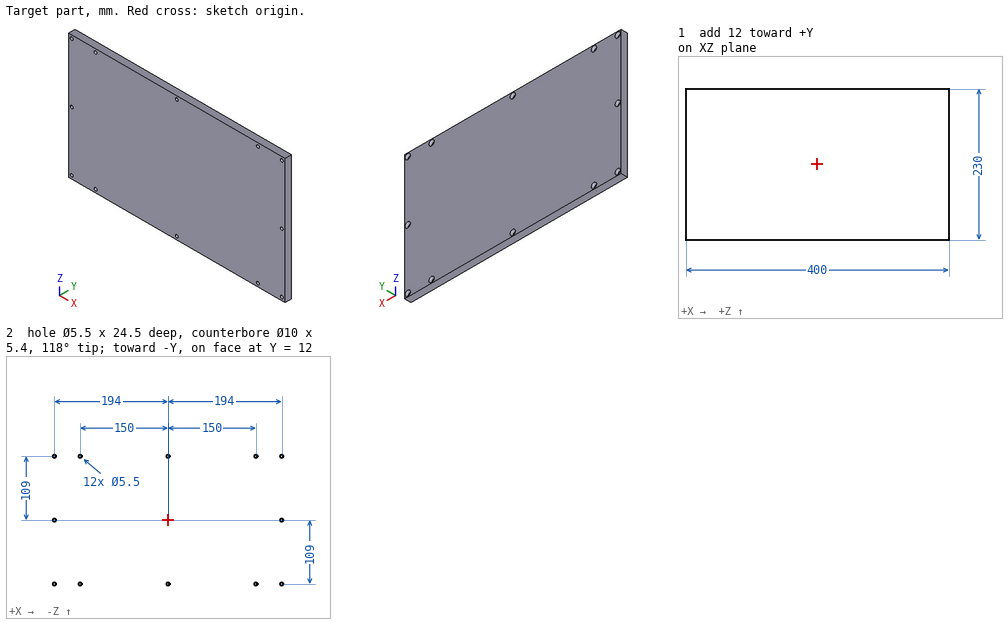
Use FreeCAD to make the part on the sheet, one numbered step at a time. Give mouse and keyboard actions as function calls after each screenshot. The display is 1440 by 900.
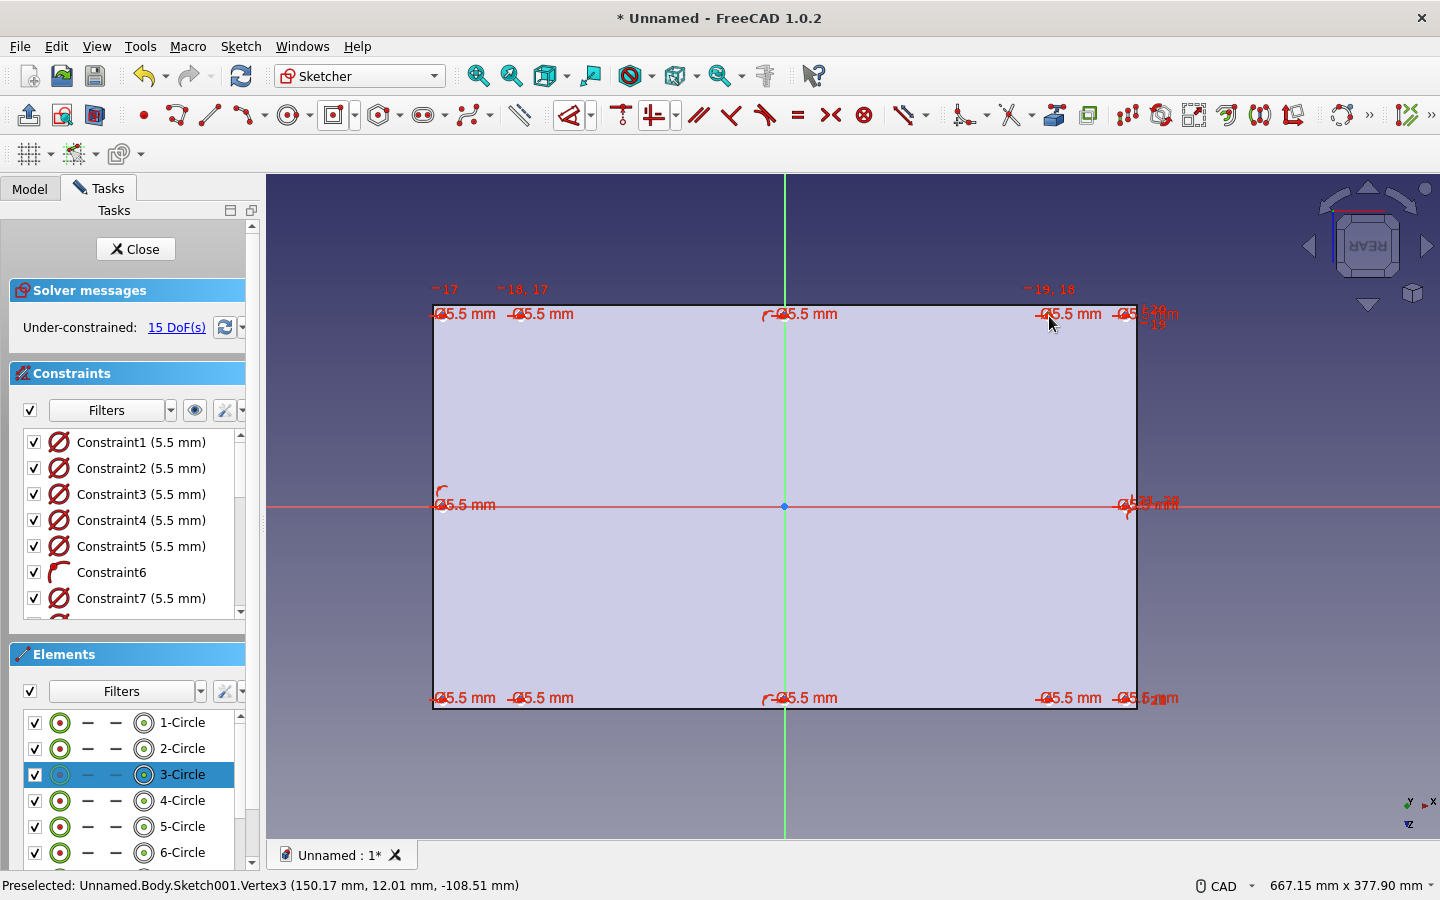
click(1049, 700)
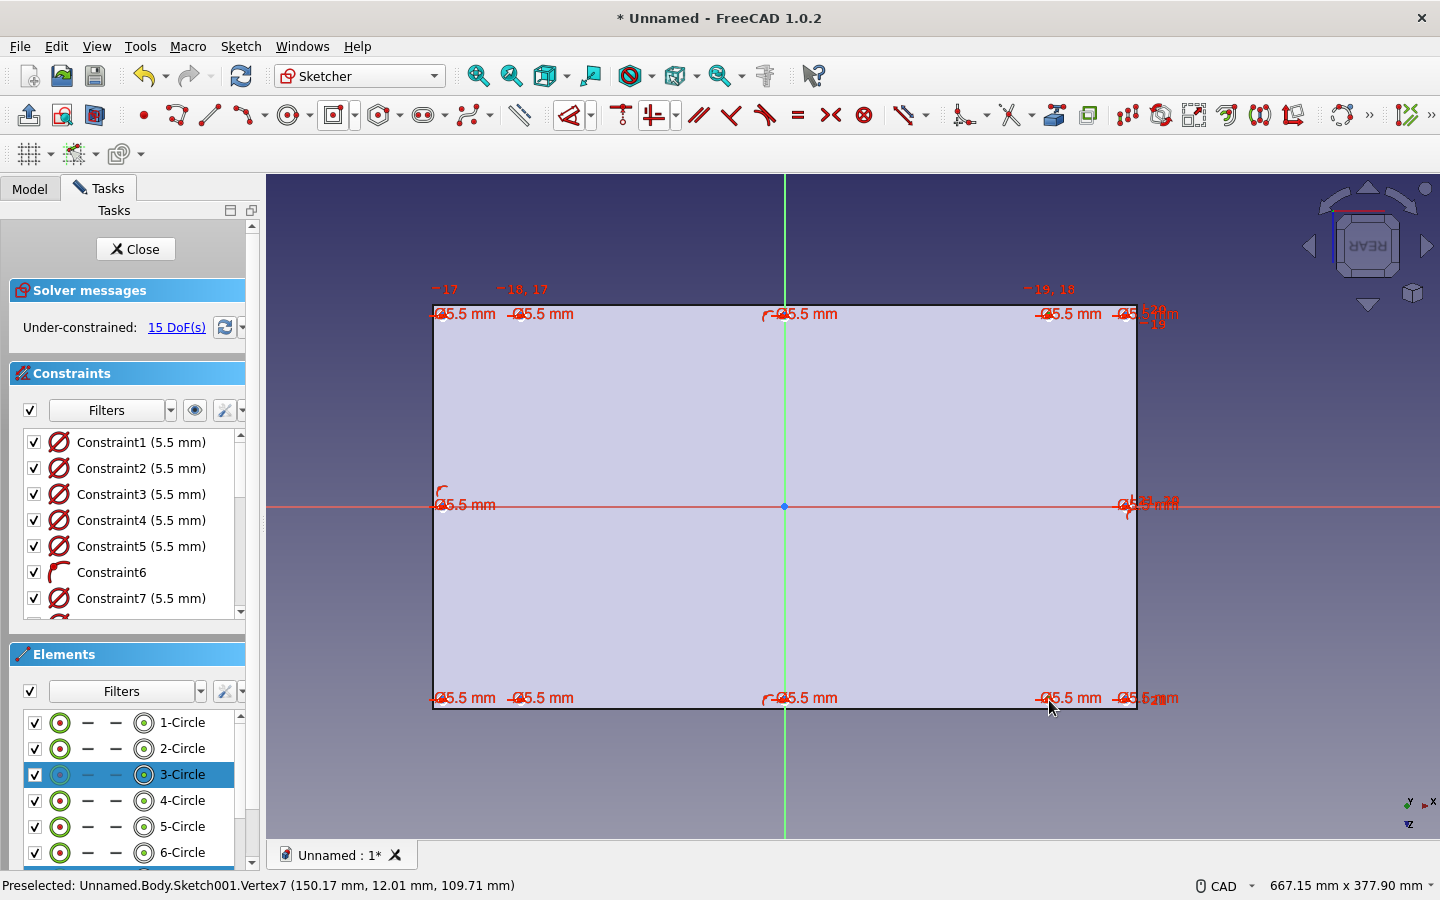
key(v)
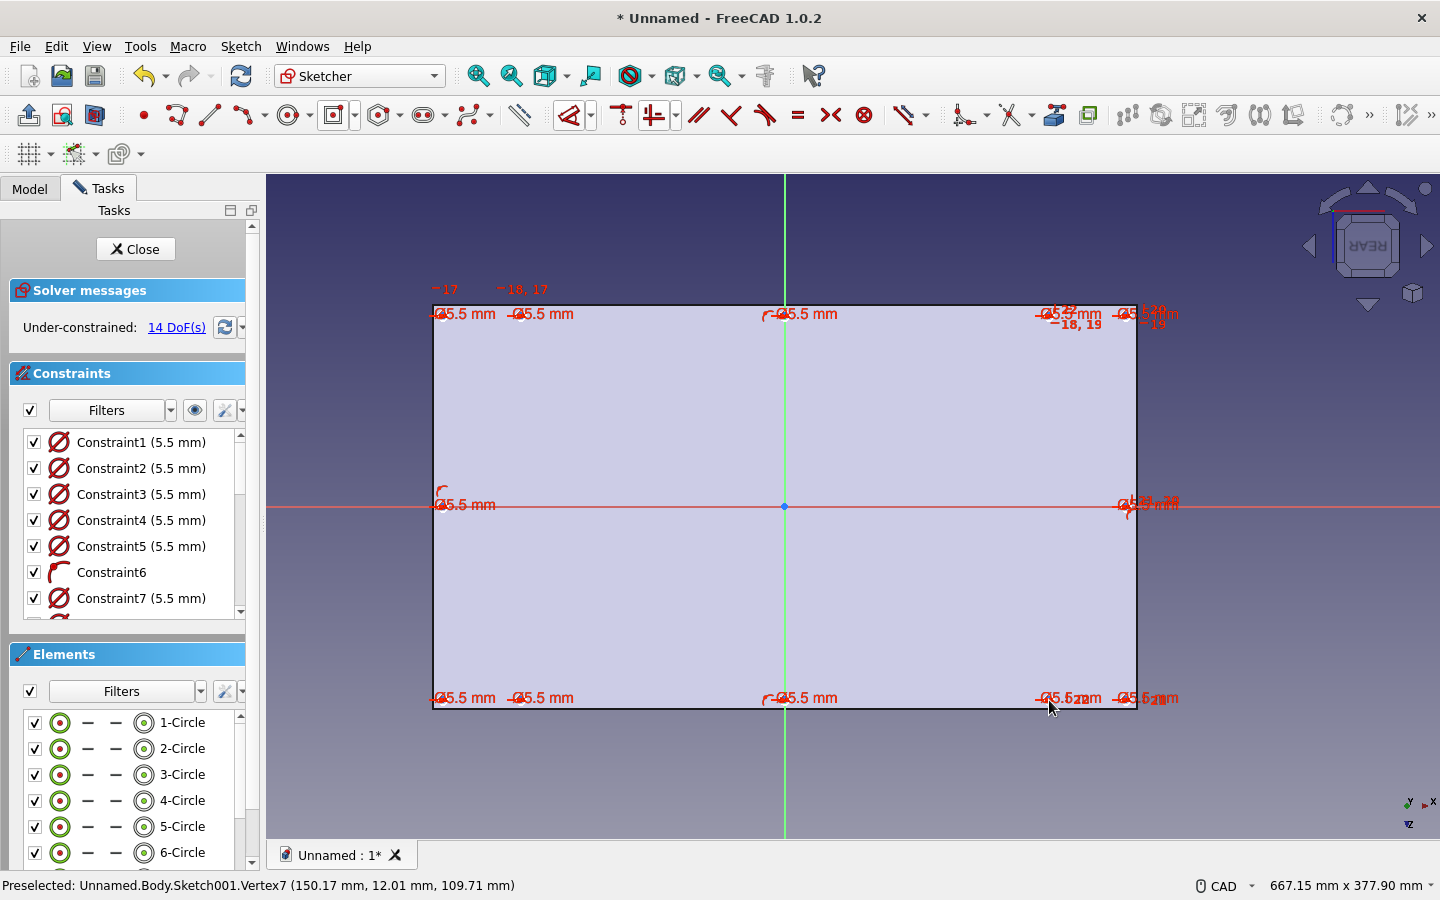
click(1126, 700)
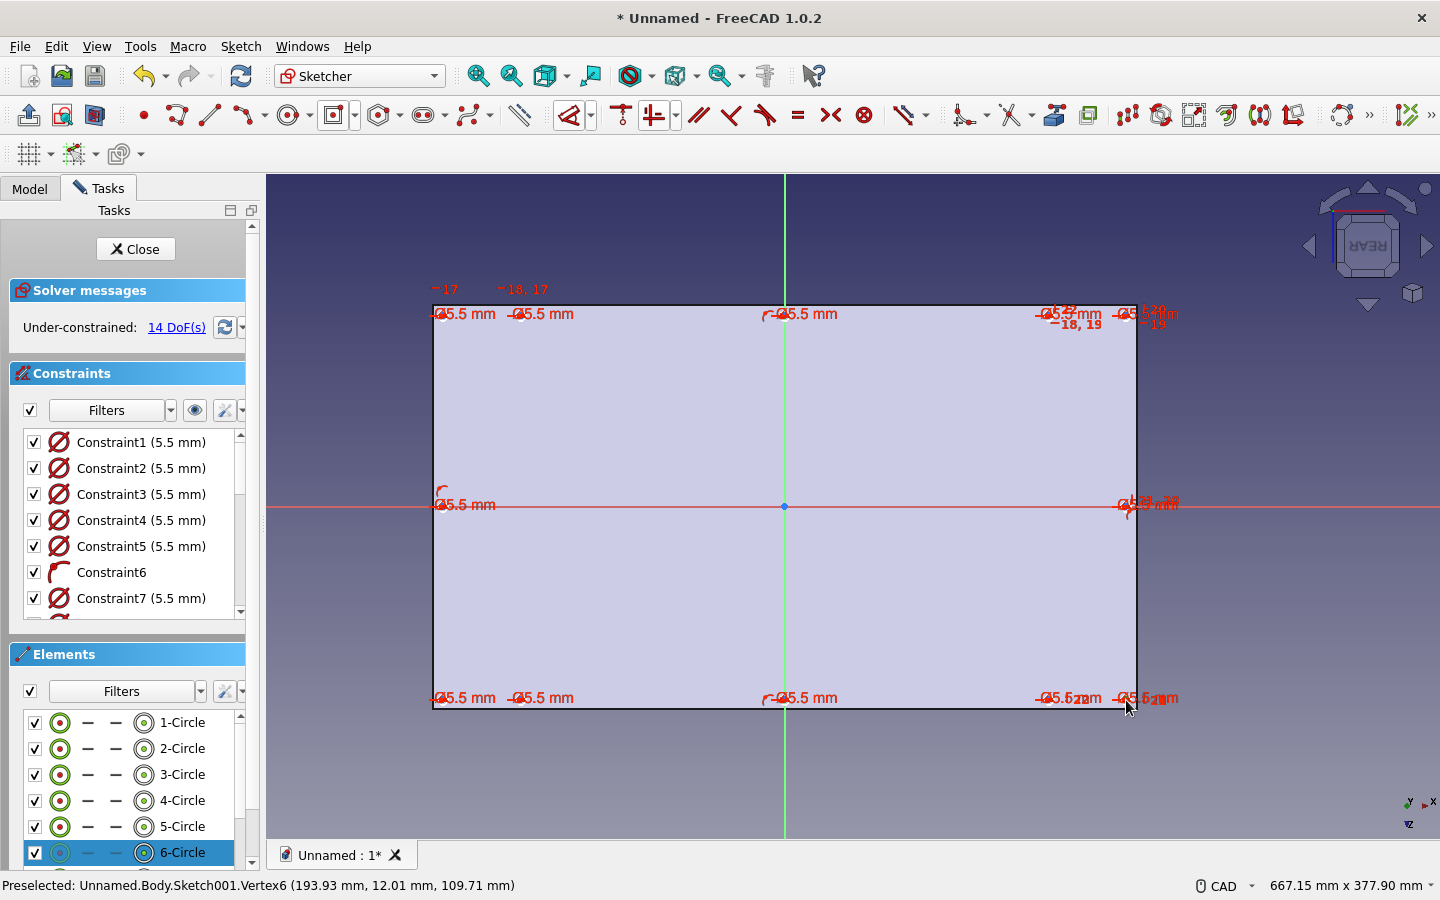
click(1049, 700)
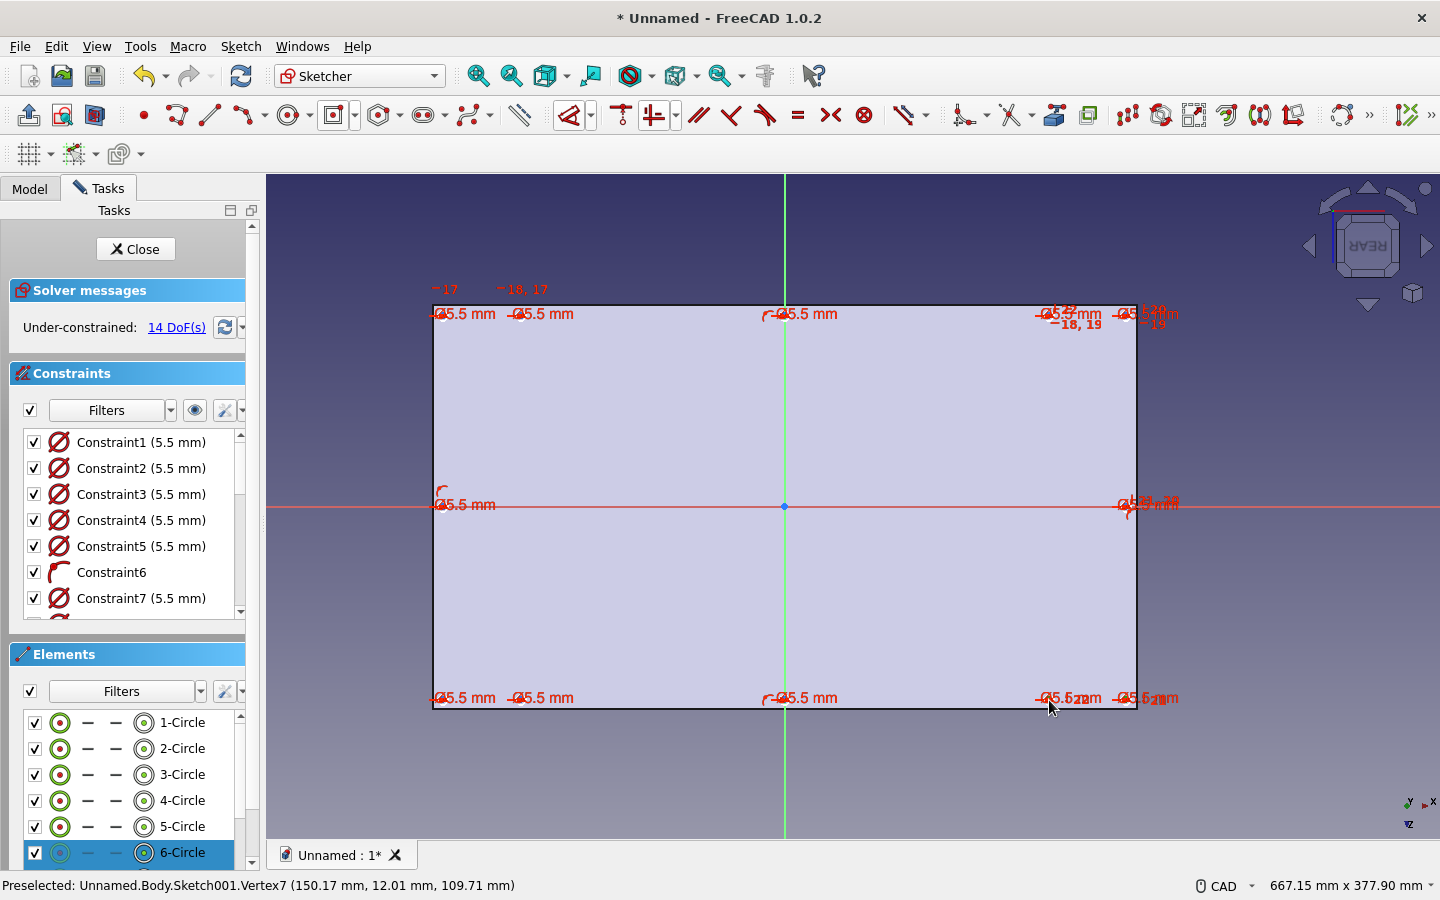
key(h)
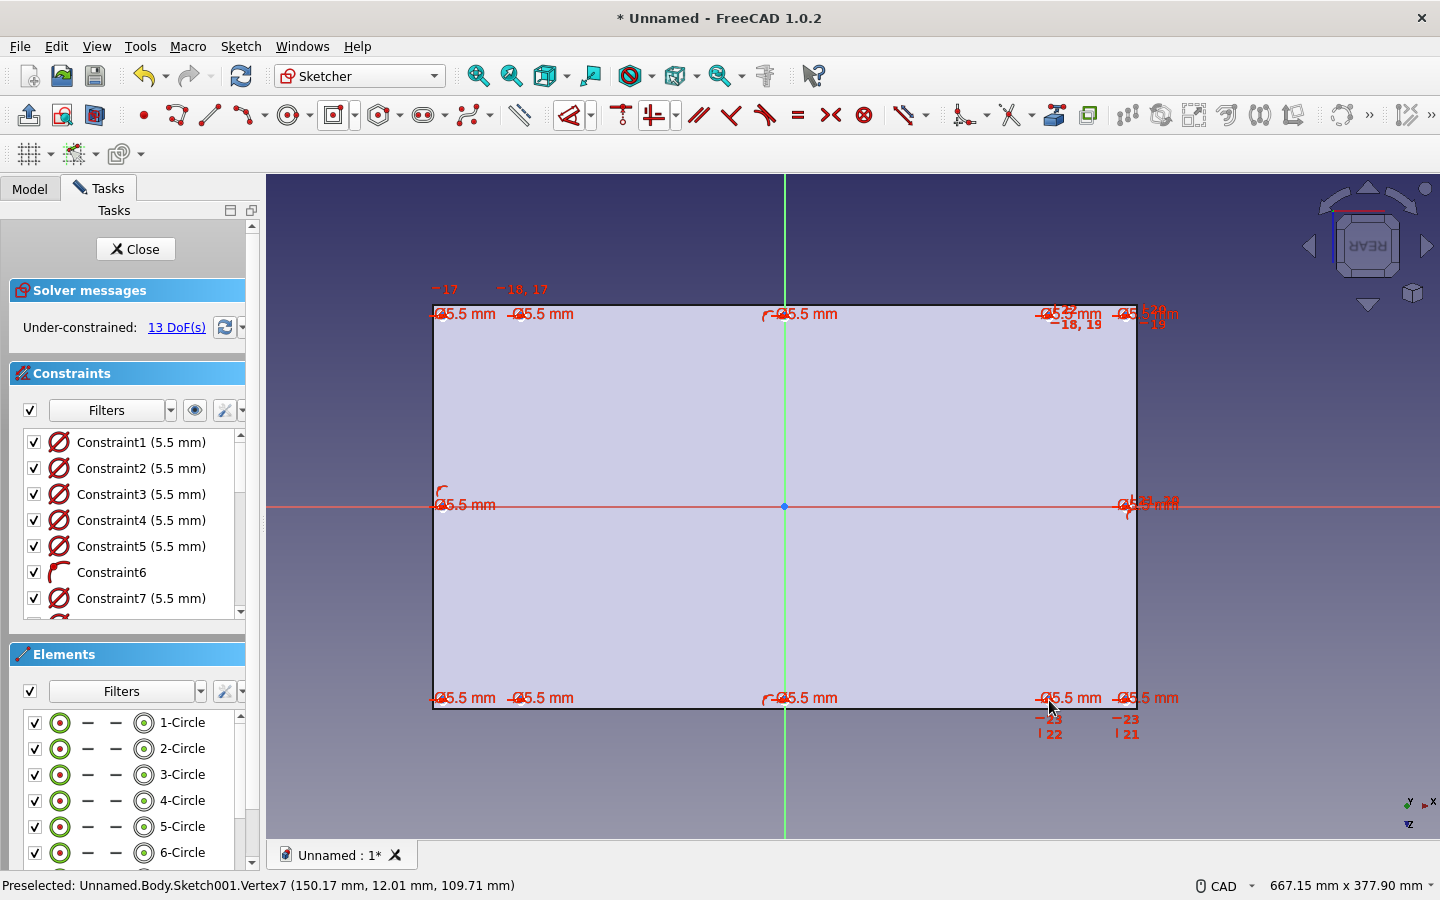
click(521, 316)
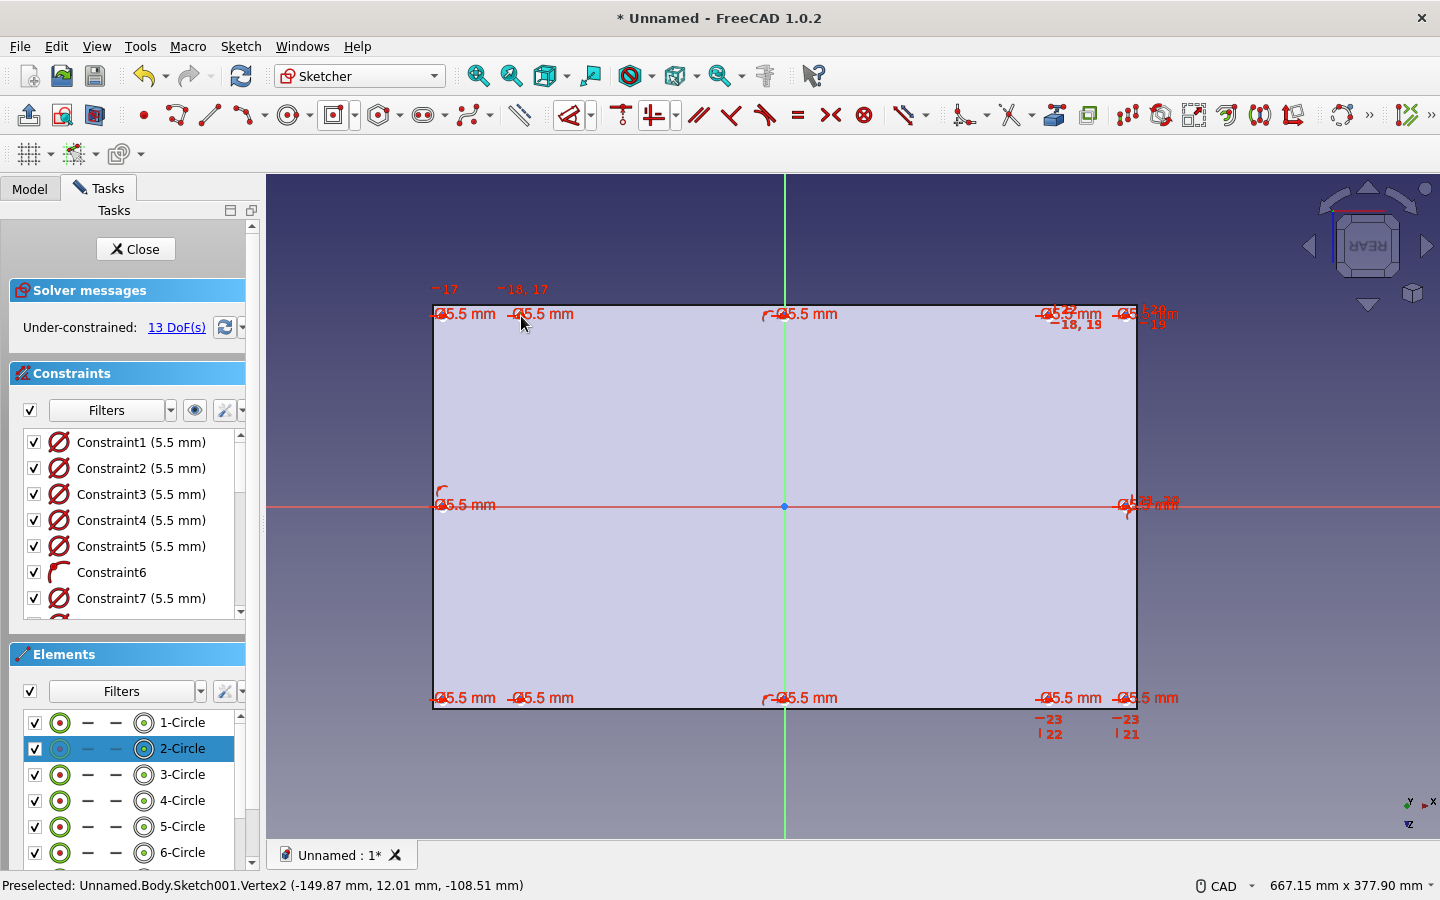
click(521, 700)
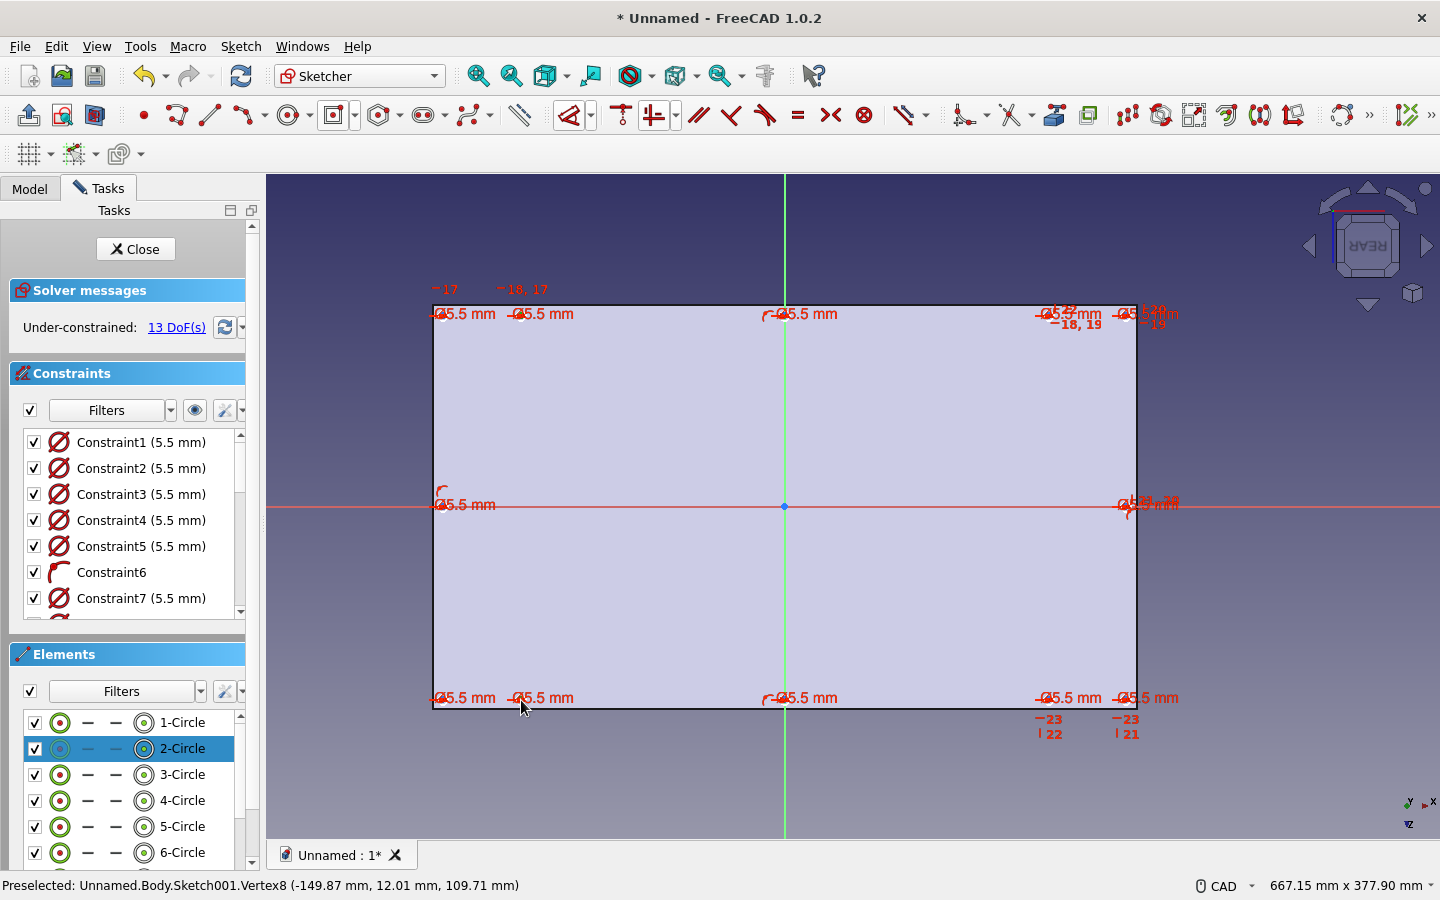
click(676, 116)